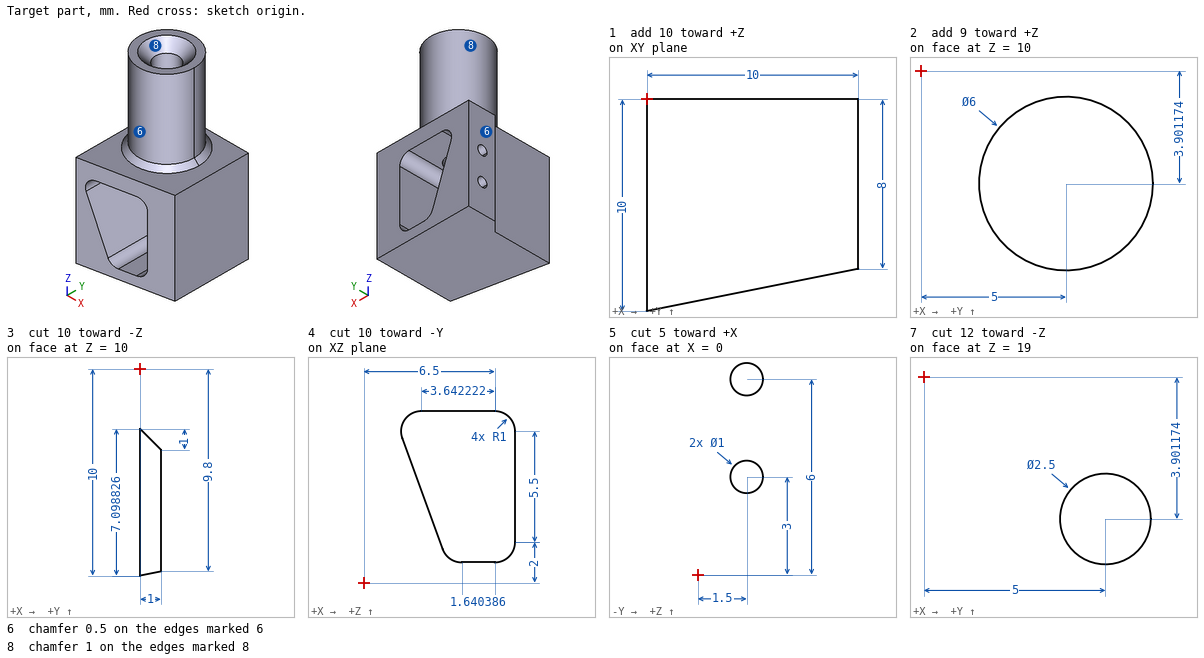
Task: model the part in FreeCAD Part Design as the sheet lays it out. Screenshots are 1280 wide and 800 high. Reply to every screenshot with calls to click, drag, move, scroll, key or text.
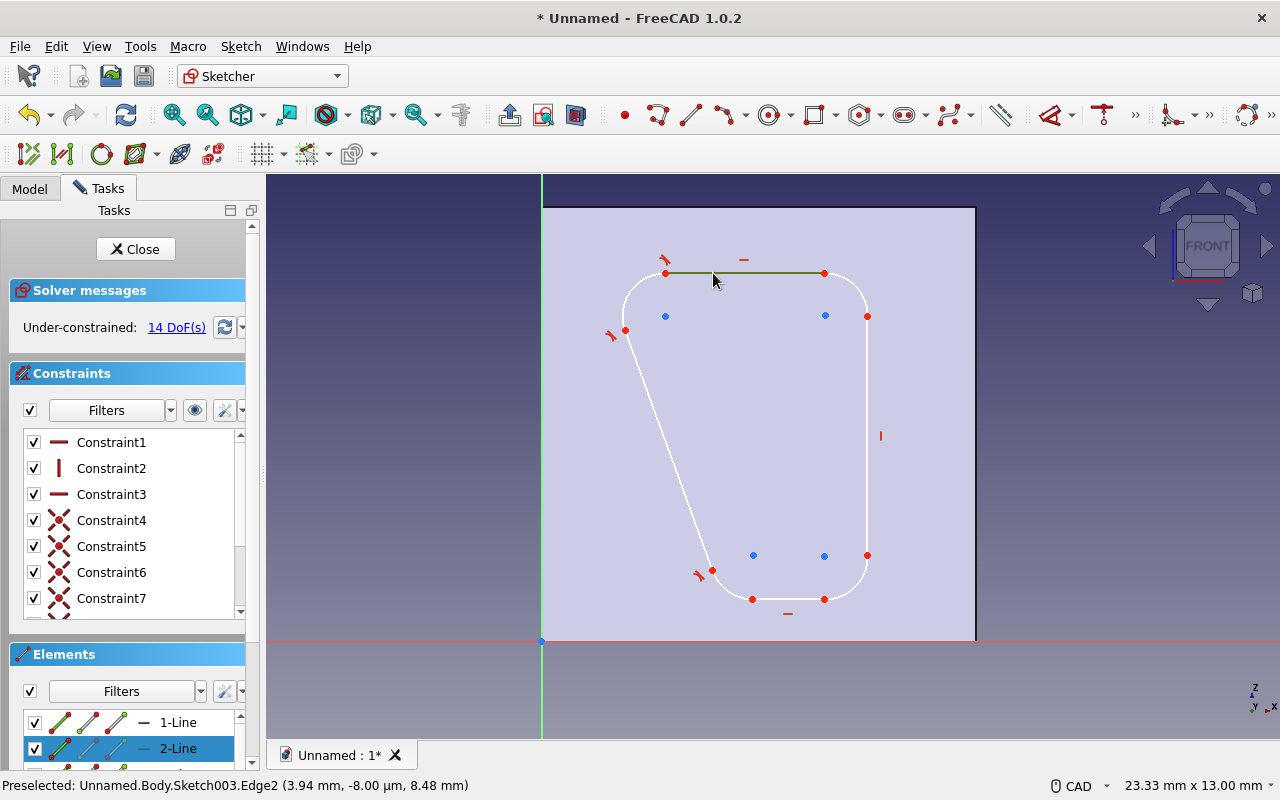
click(863, 297)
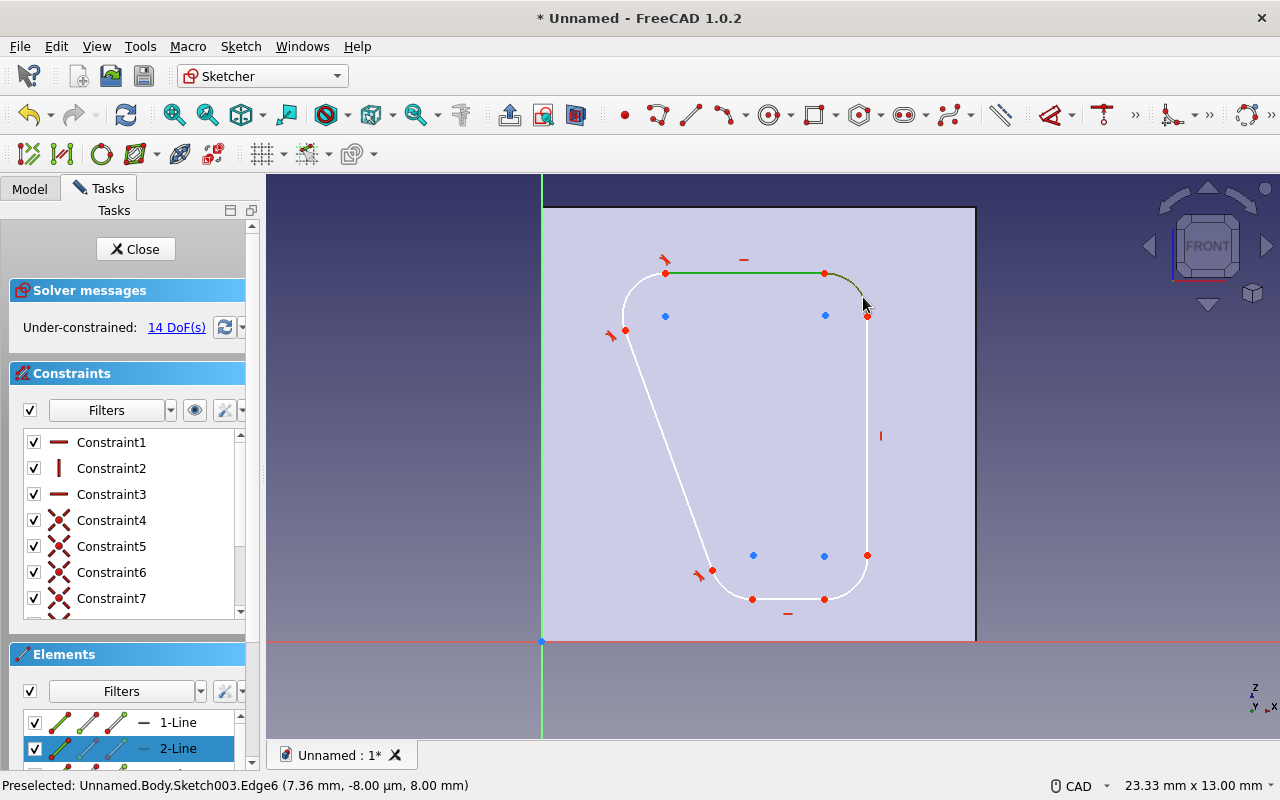
key(t)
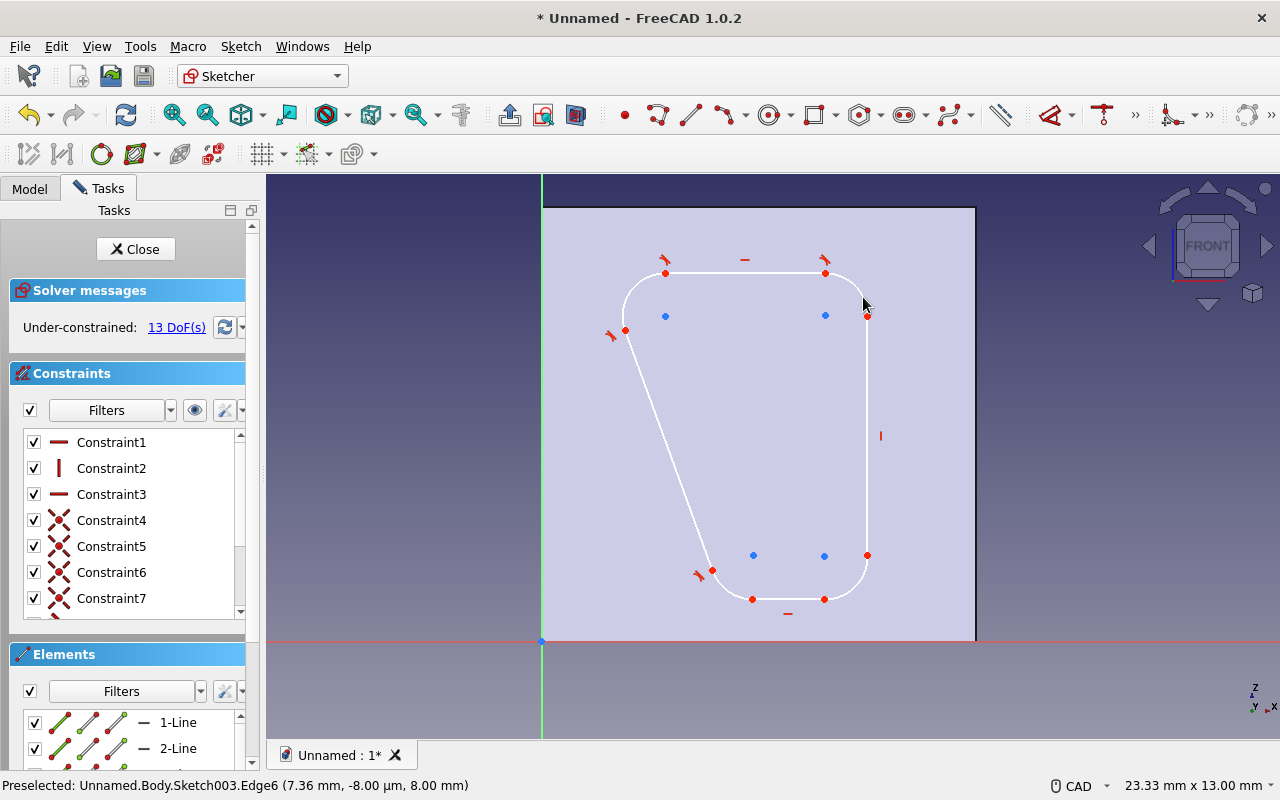
click(867, 388)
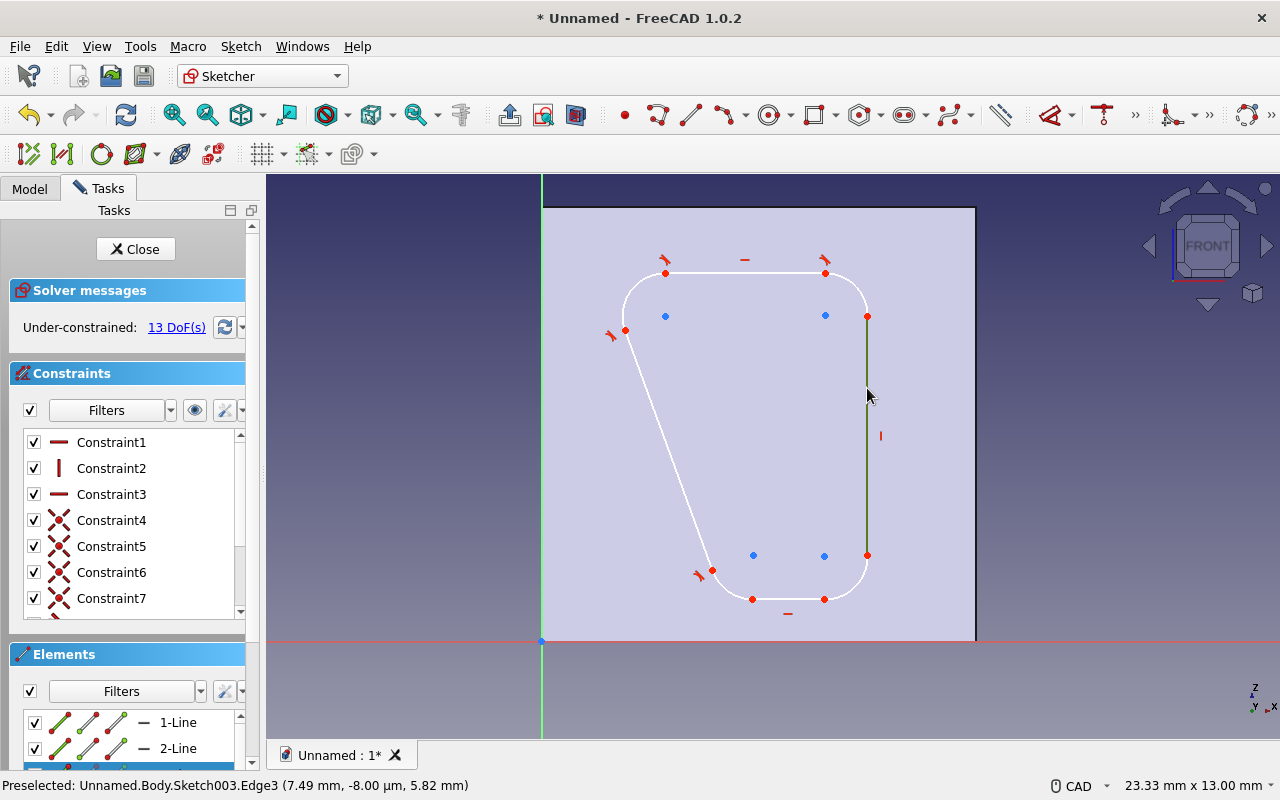
click(863, 297)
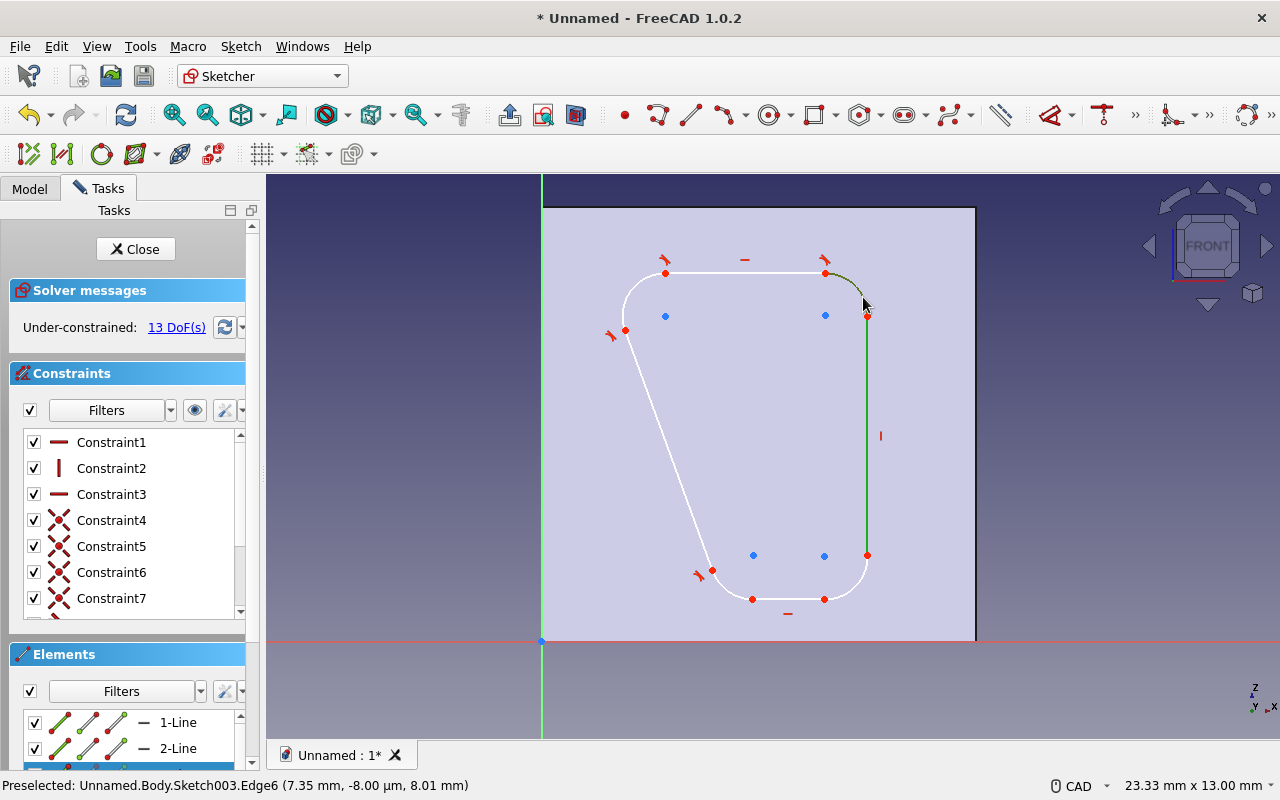
key(t)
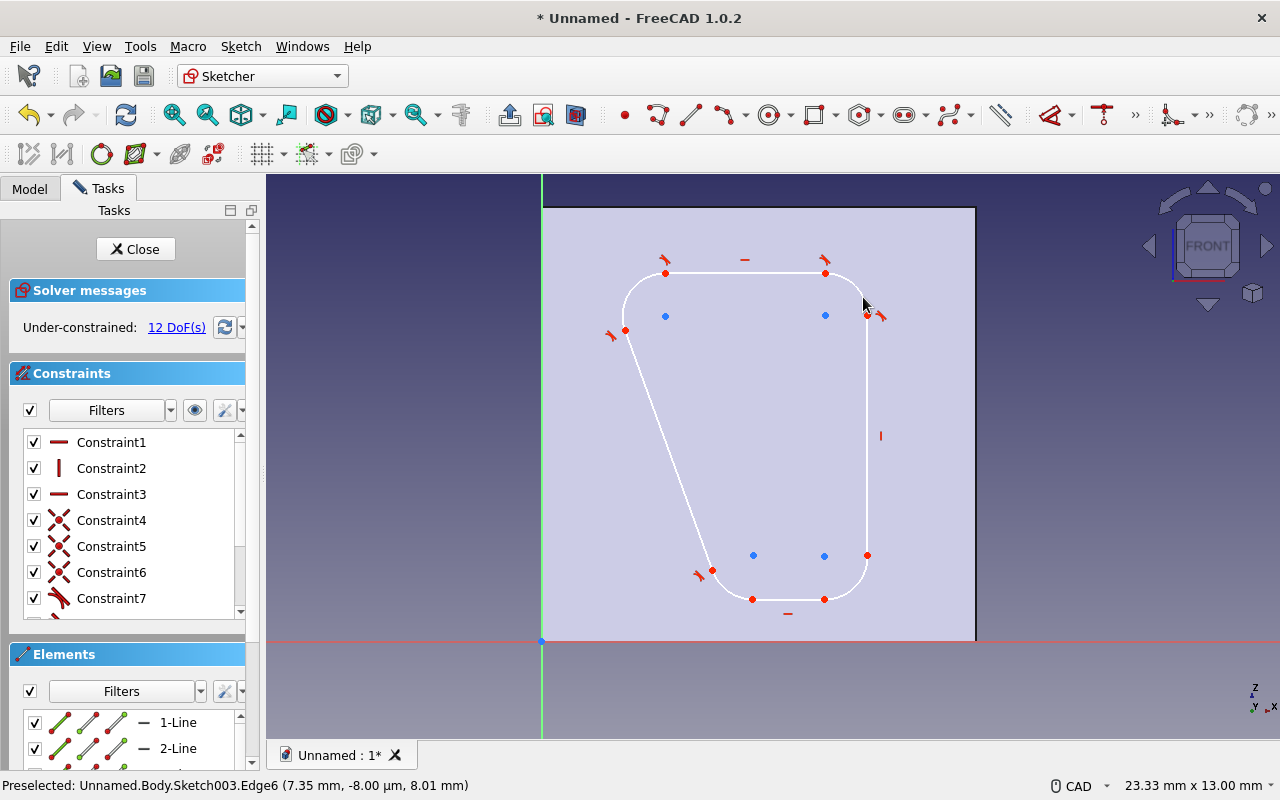
click(867, 387)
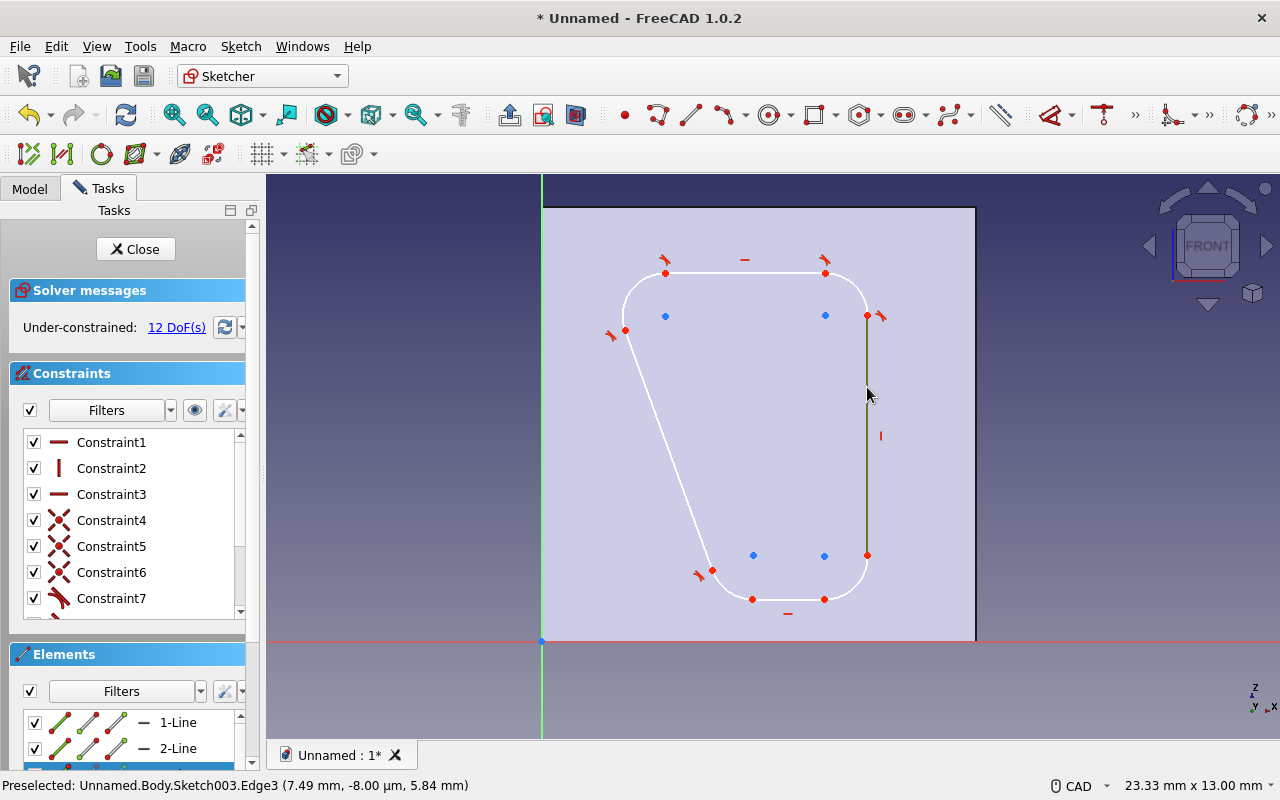
click(844, 595)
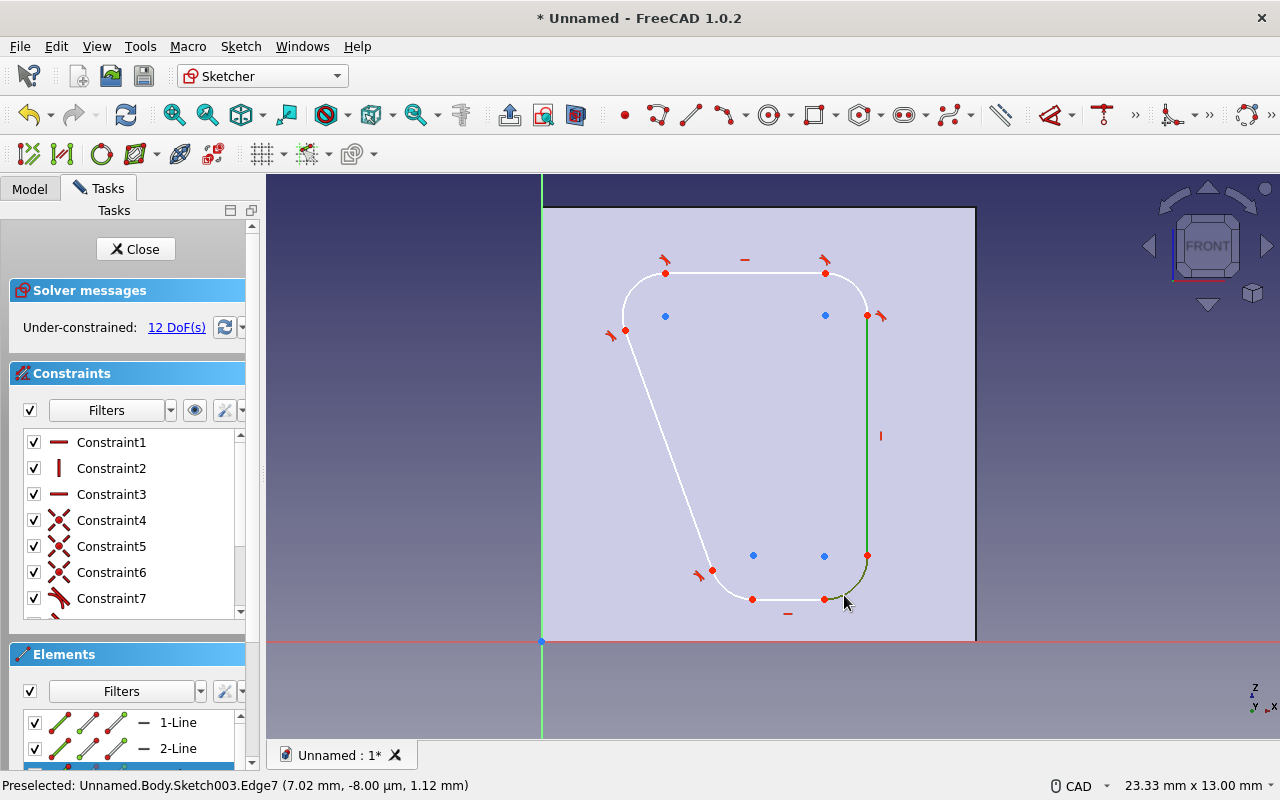
key(t)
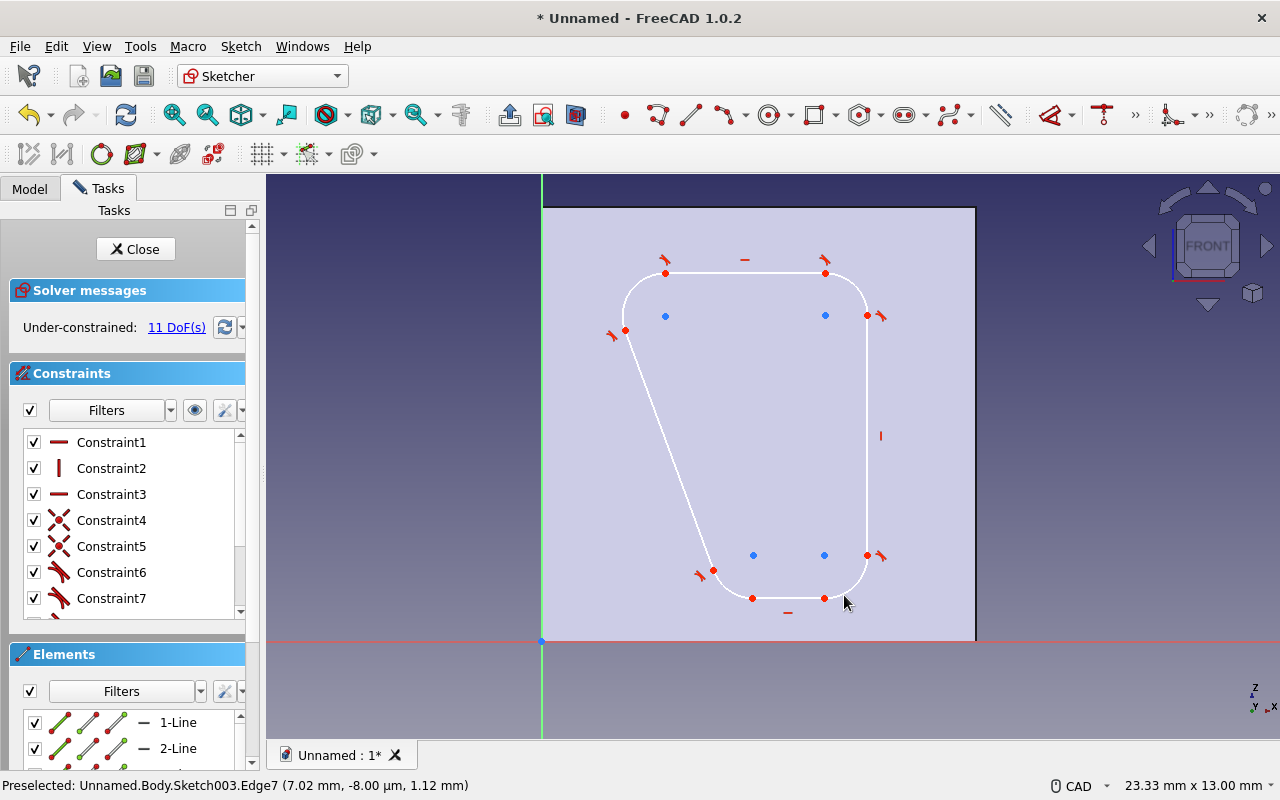
click(803, 598)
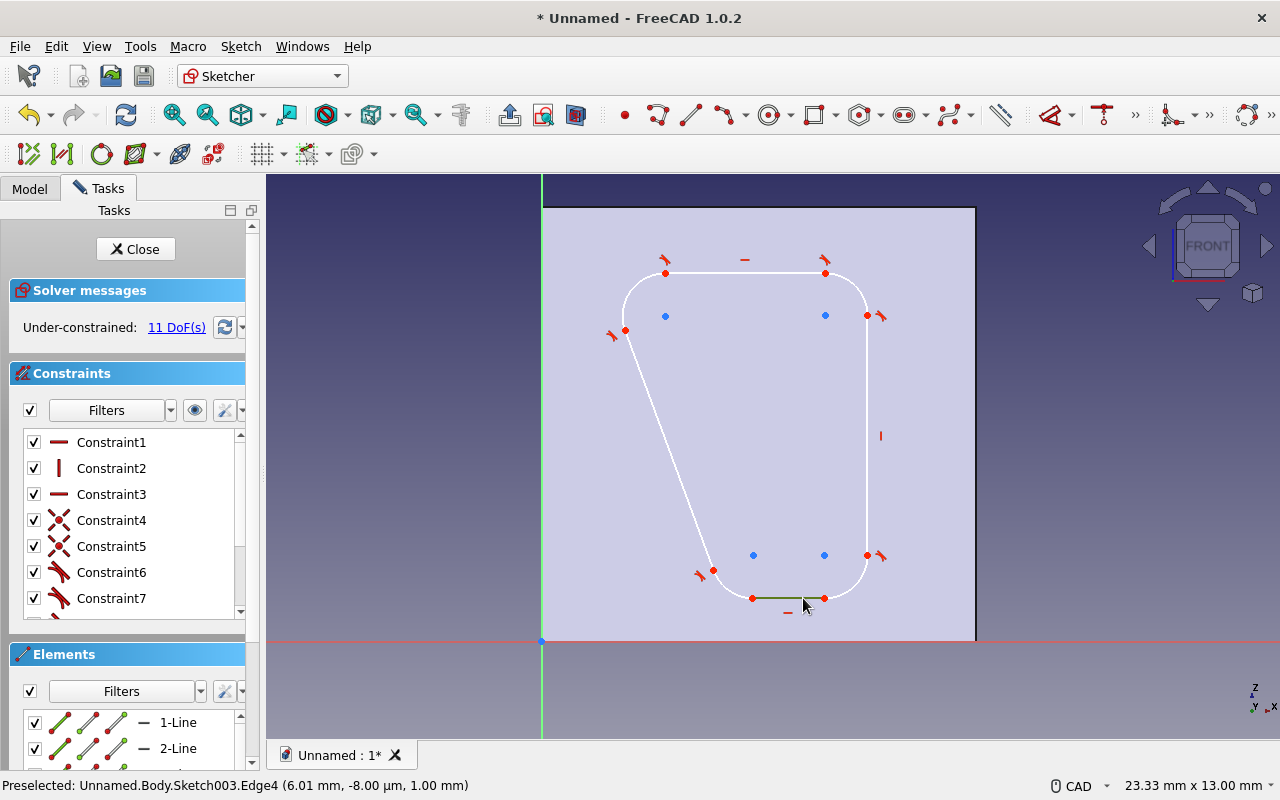
click(844, 594)